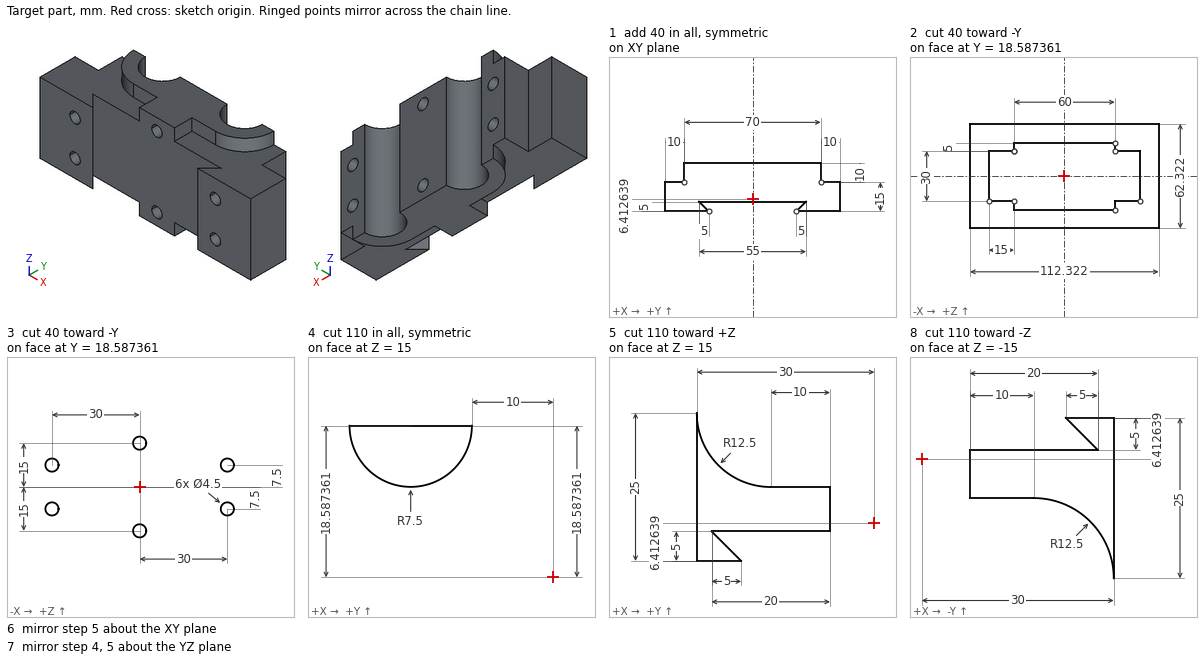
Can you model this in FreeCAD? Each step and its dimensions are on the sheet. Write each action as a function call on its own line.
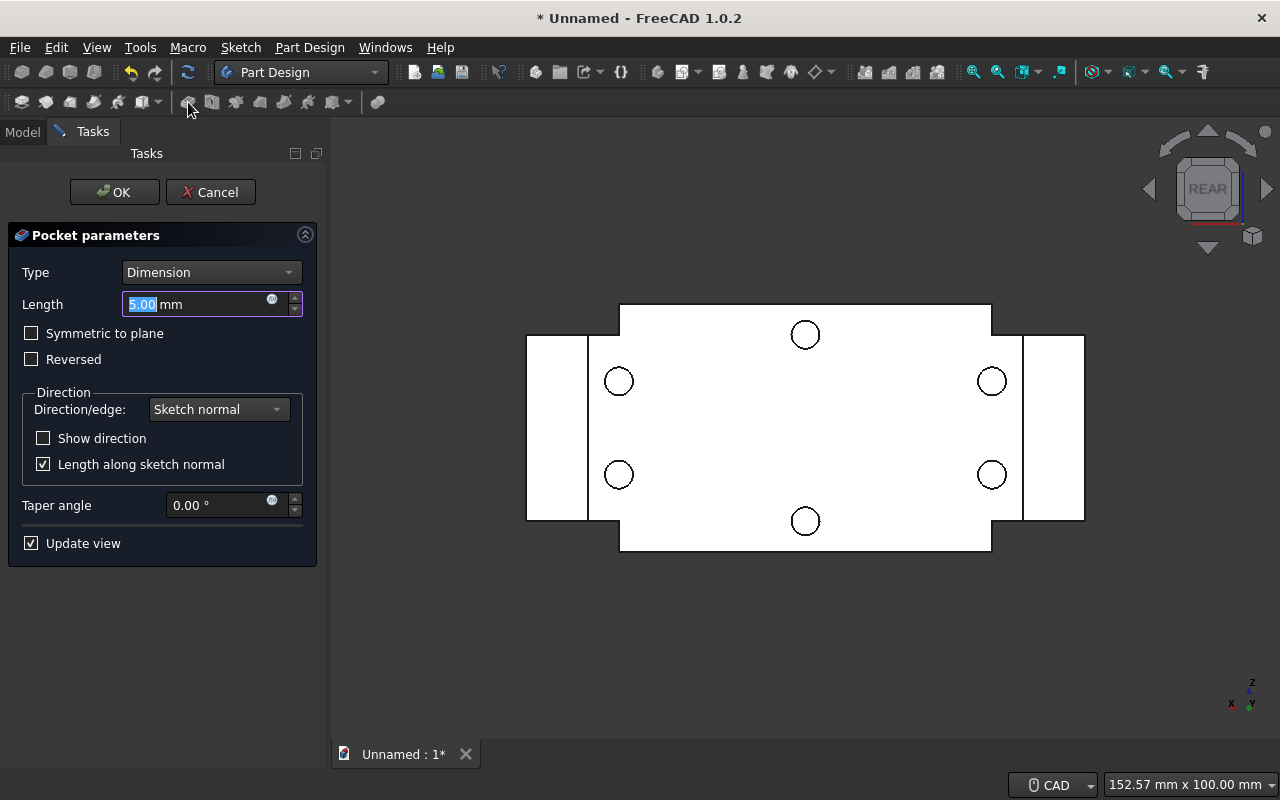
text(40)
key(Tab)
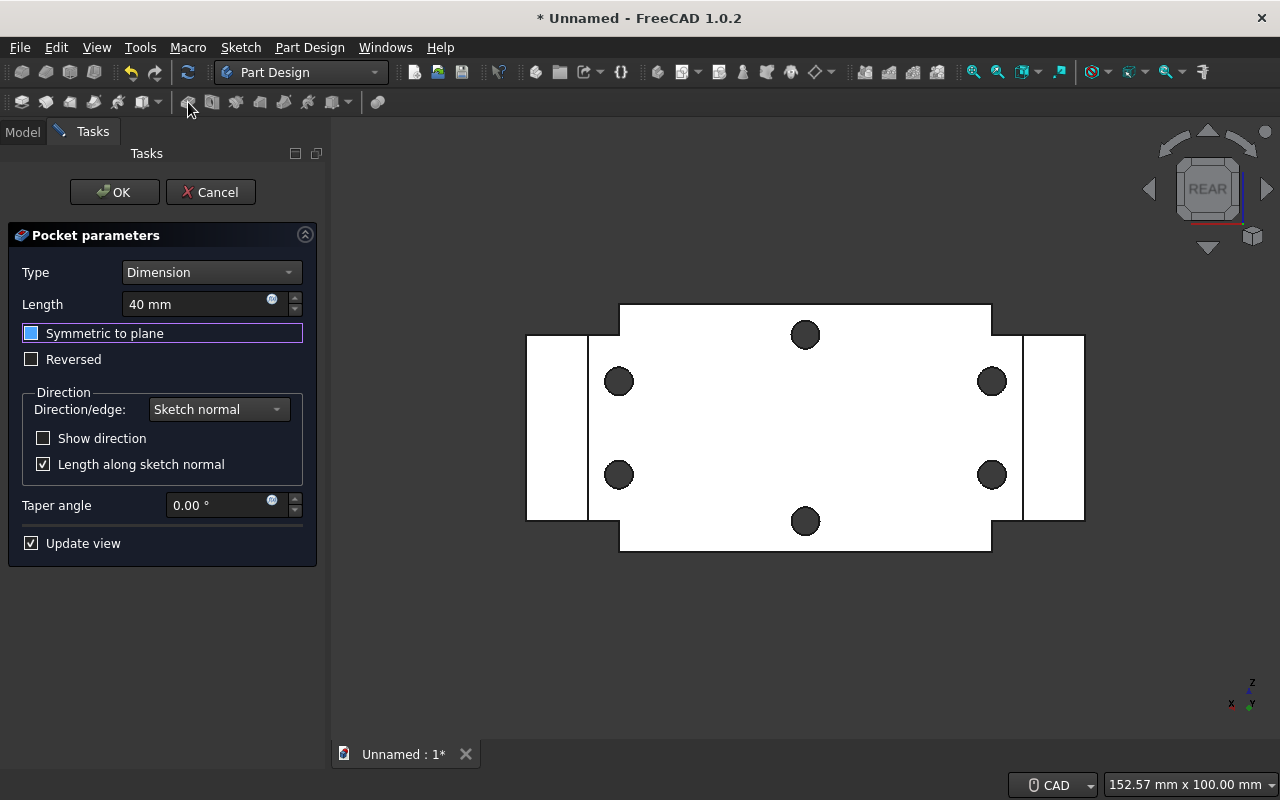
click(115, 192)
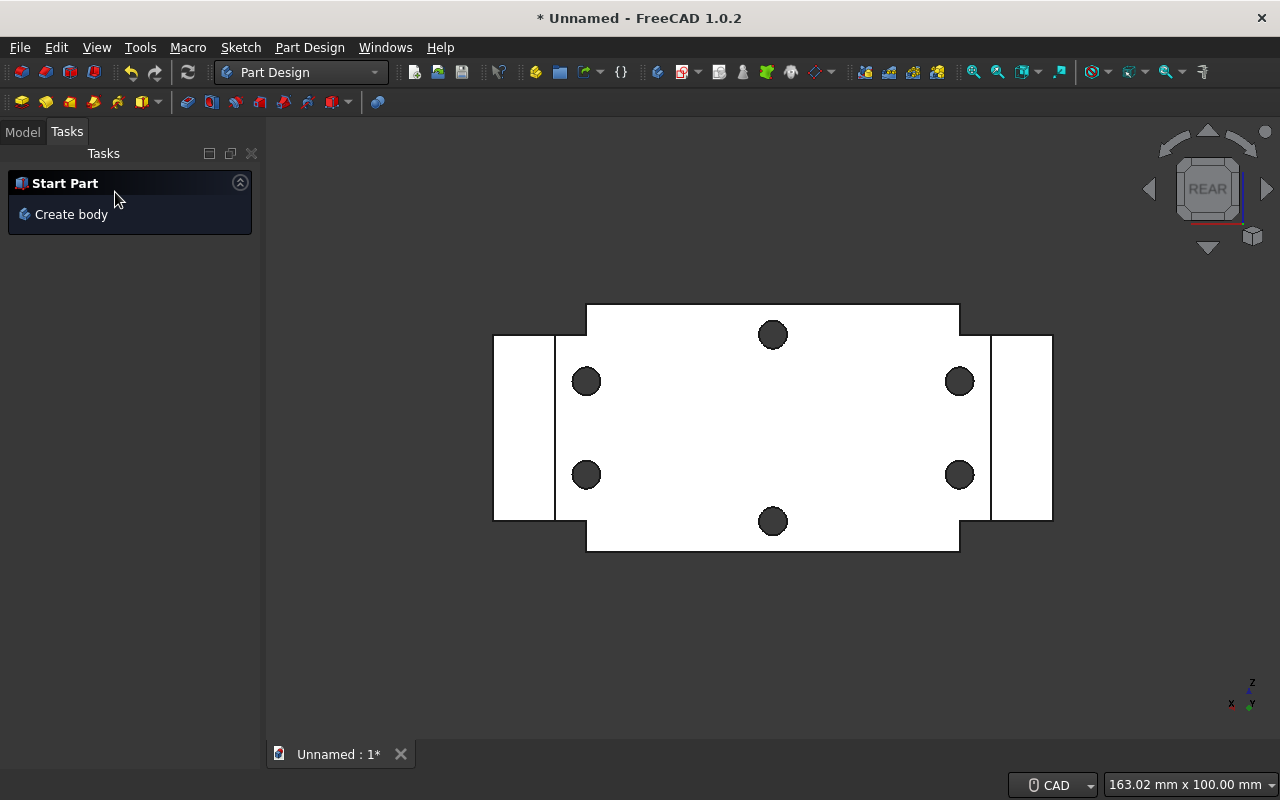
key(0)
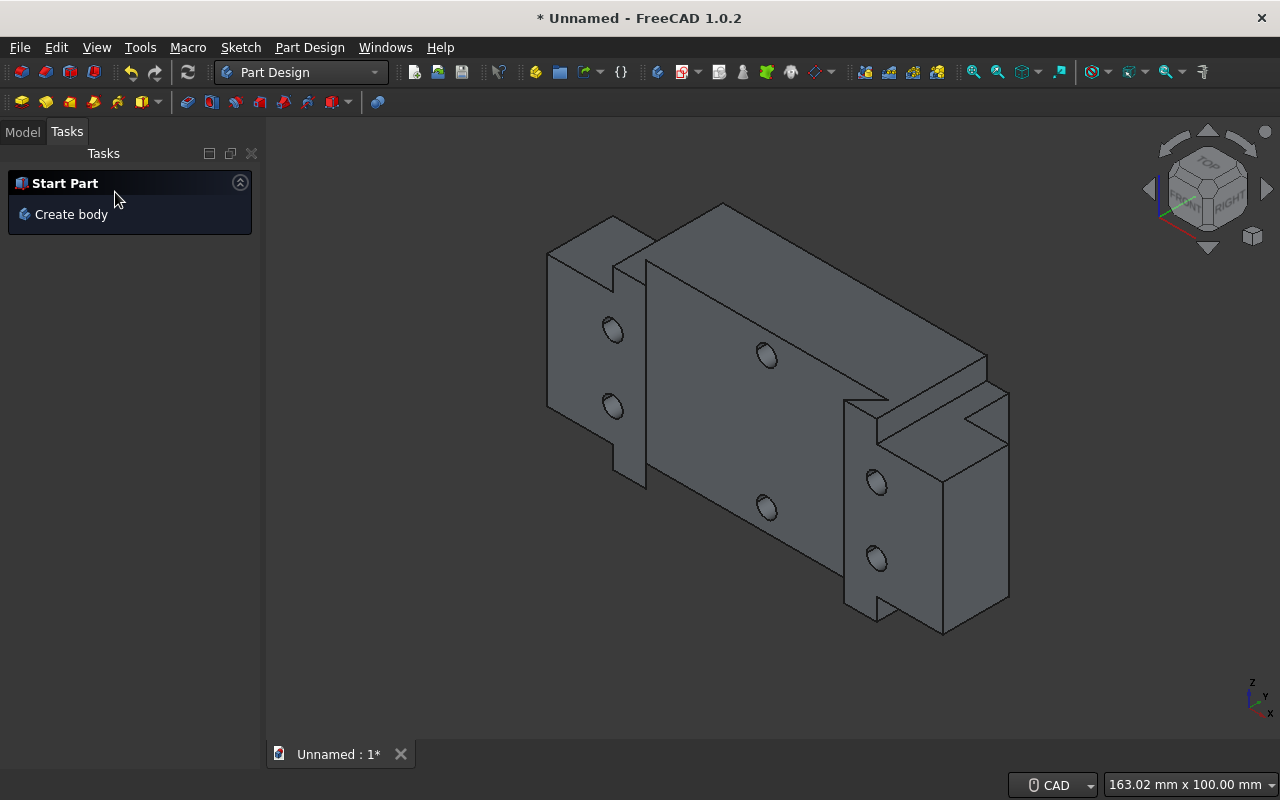
click(949, 440)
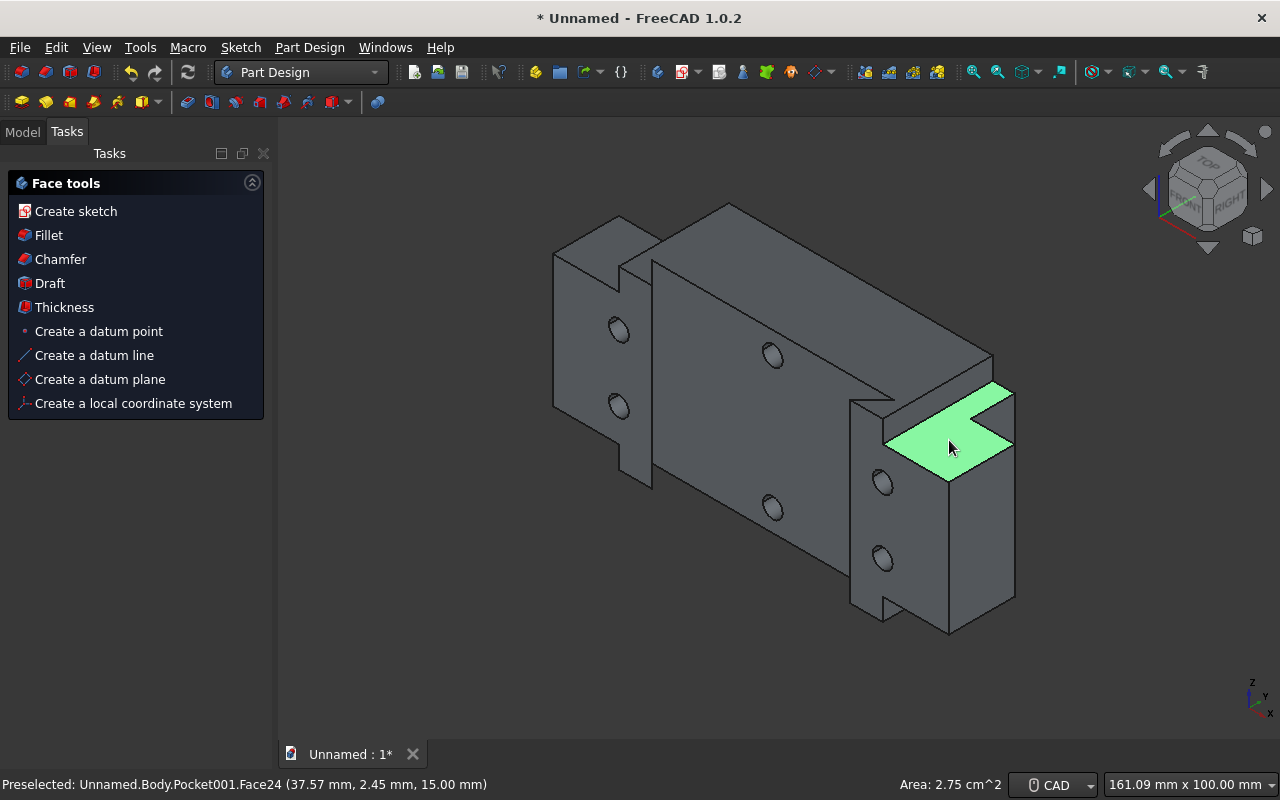
click(682, 72)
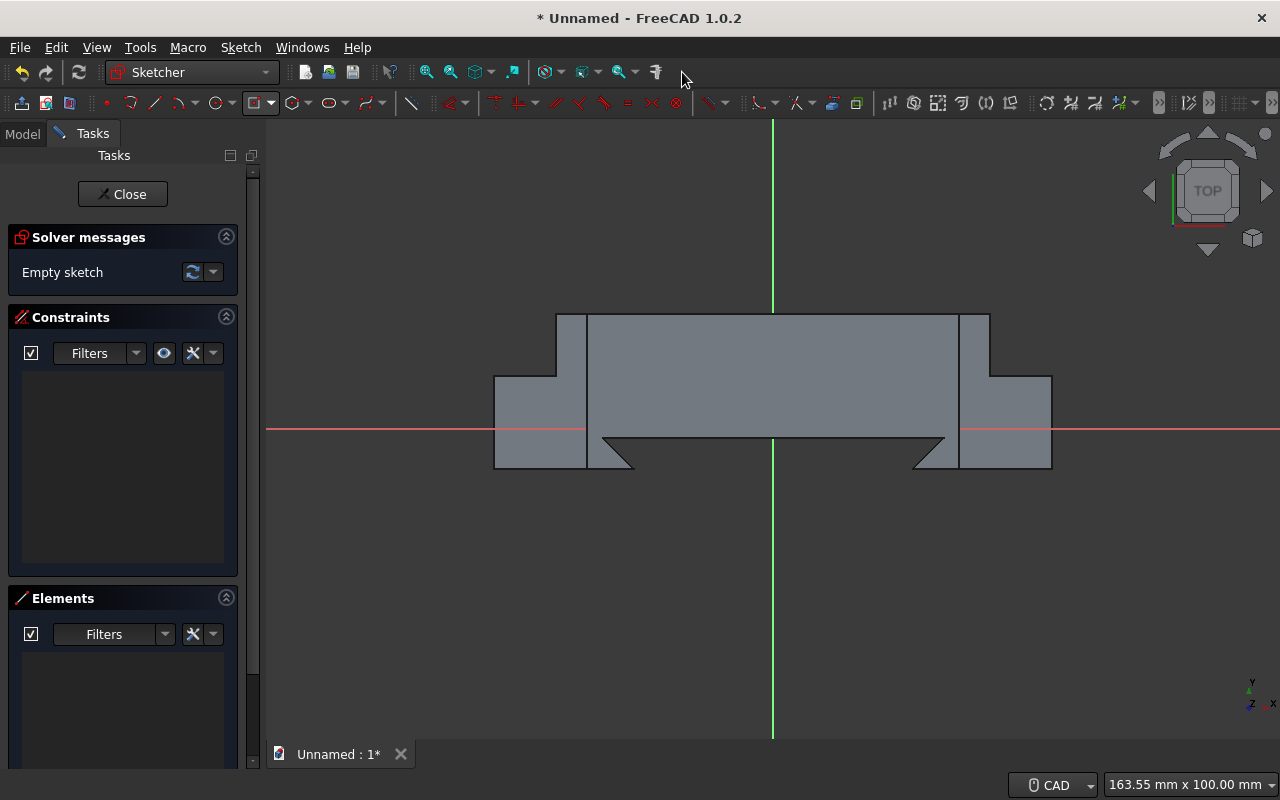
key(q)
key(s)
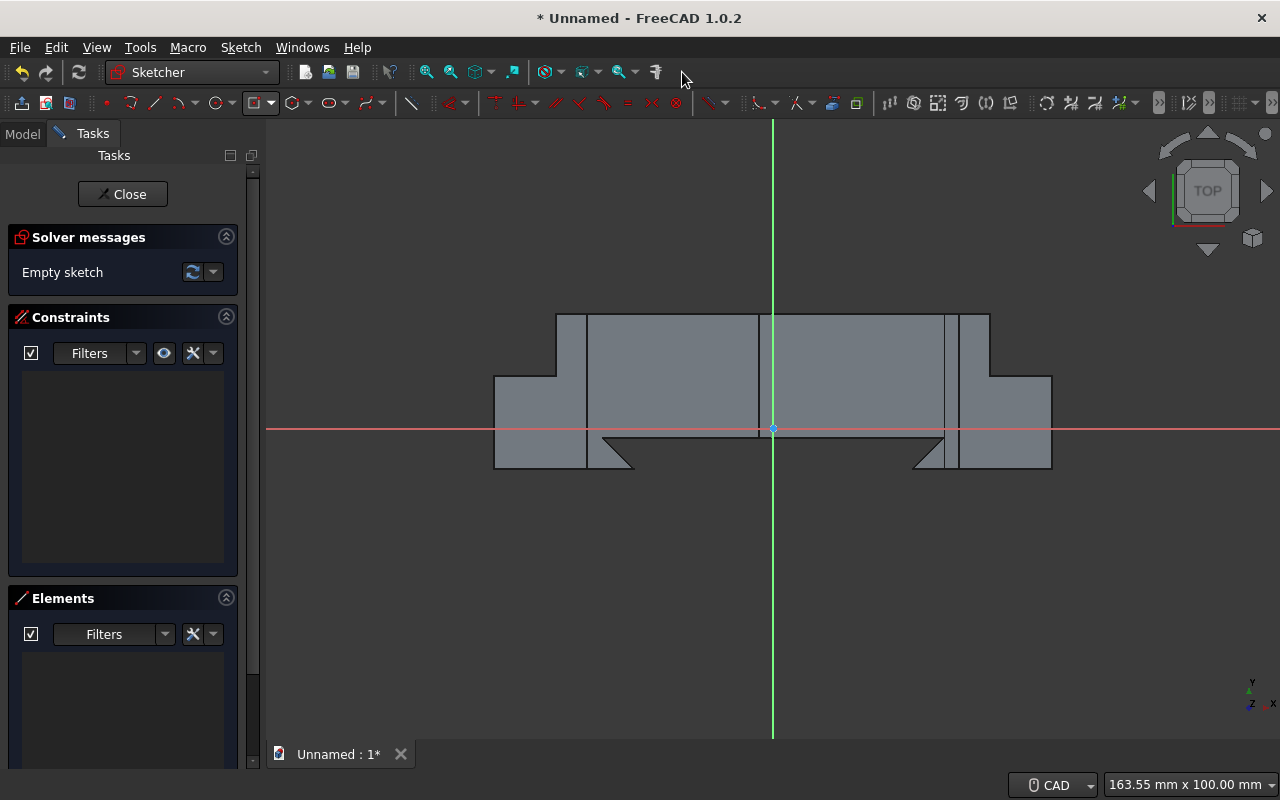
scroll(692, 347, up, 6)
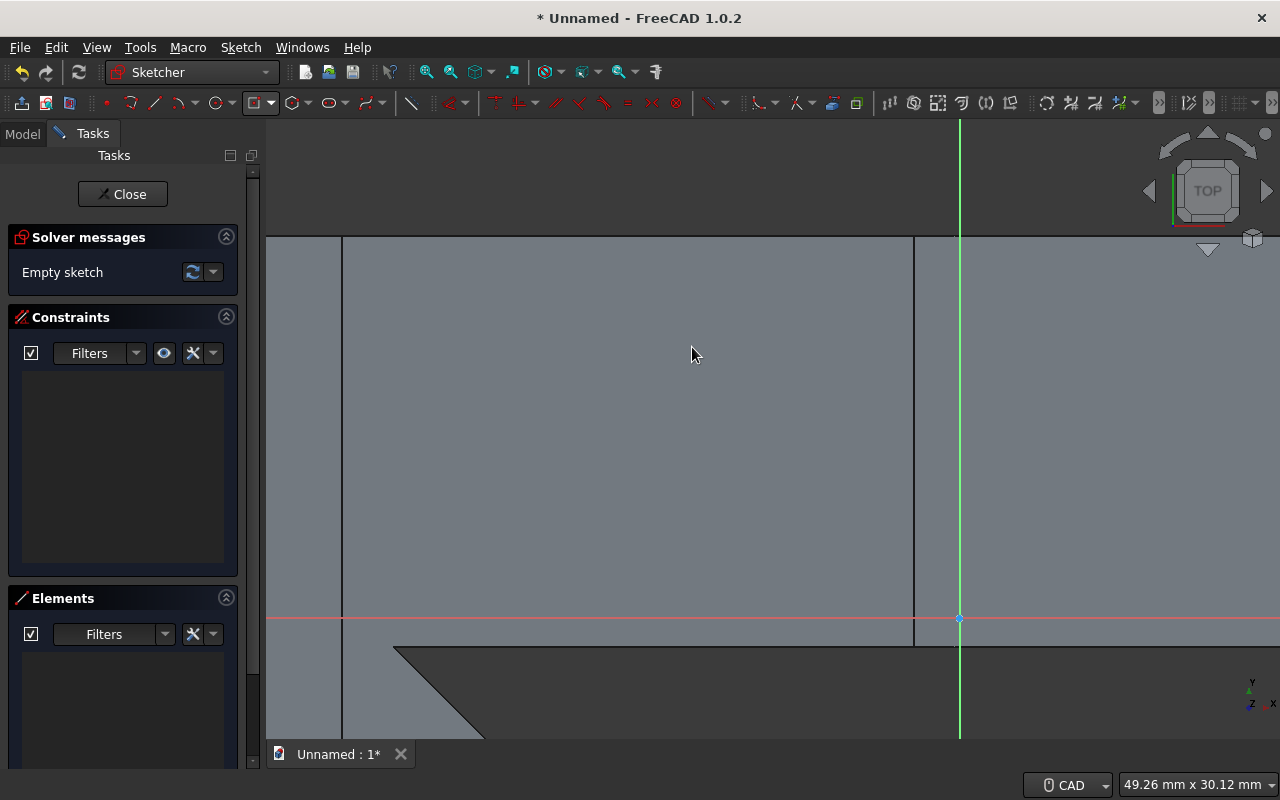
key(g)
key(l)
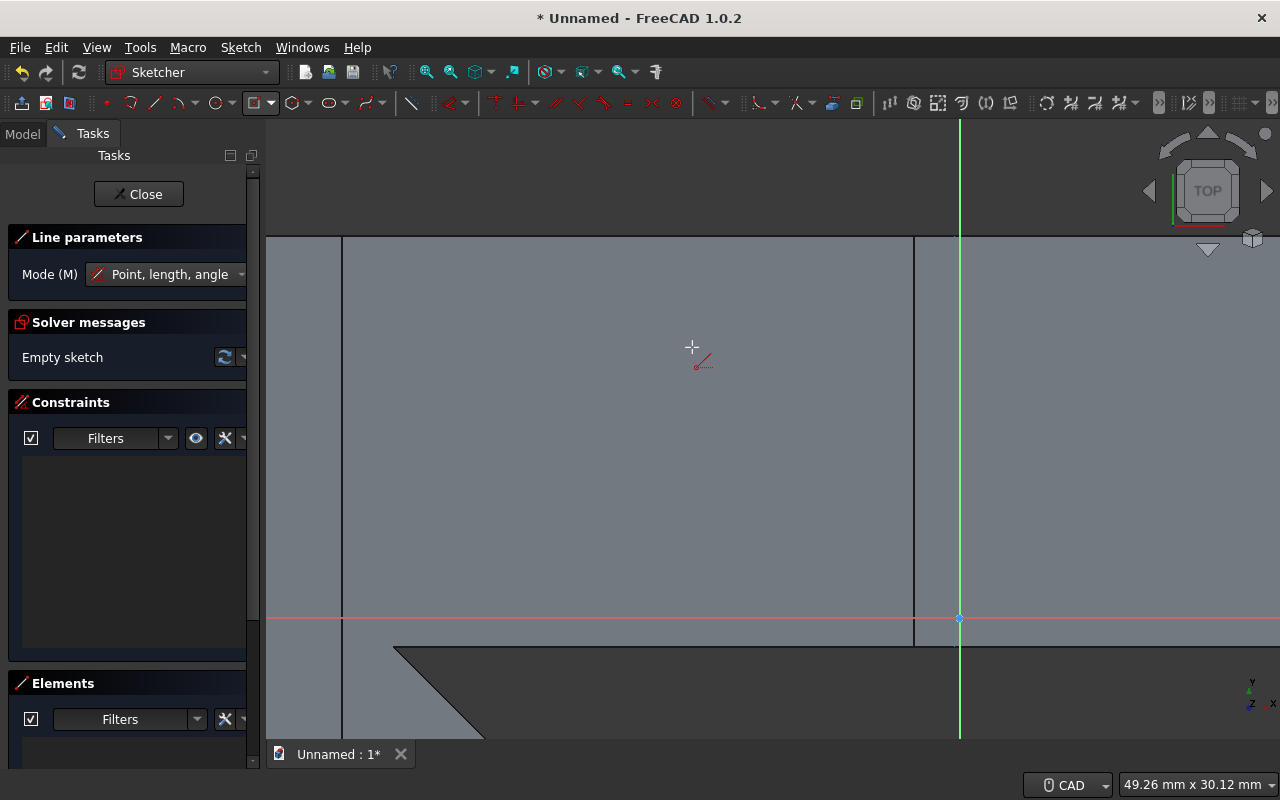
click(754, 236)
click(445, 236)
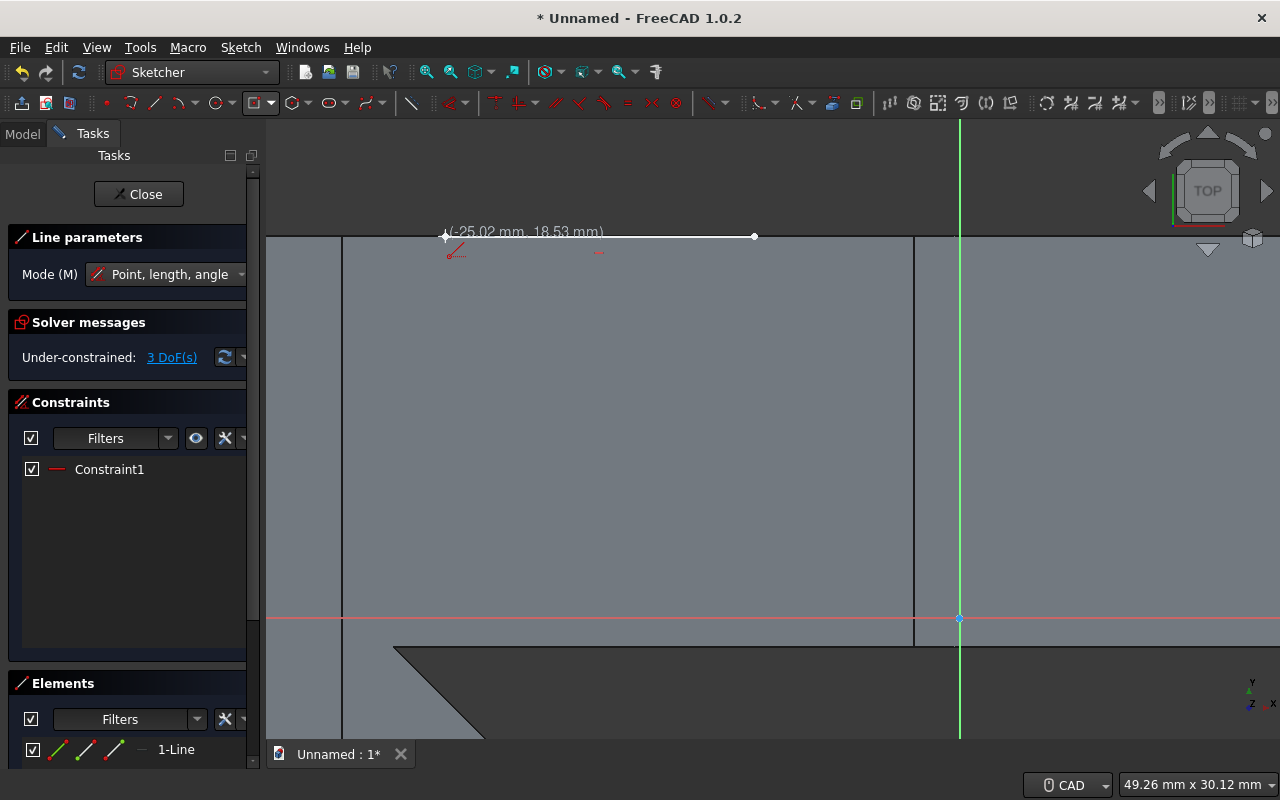
key(g)
key(3)
key(a)